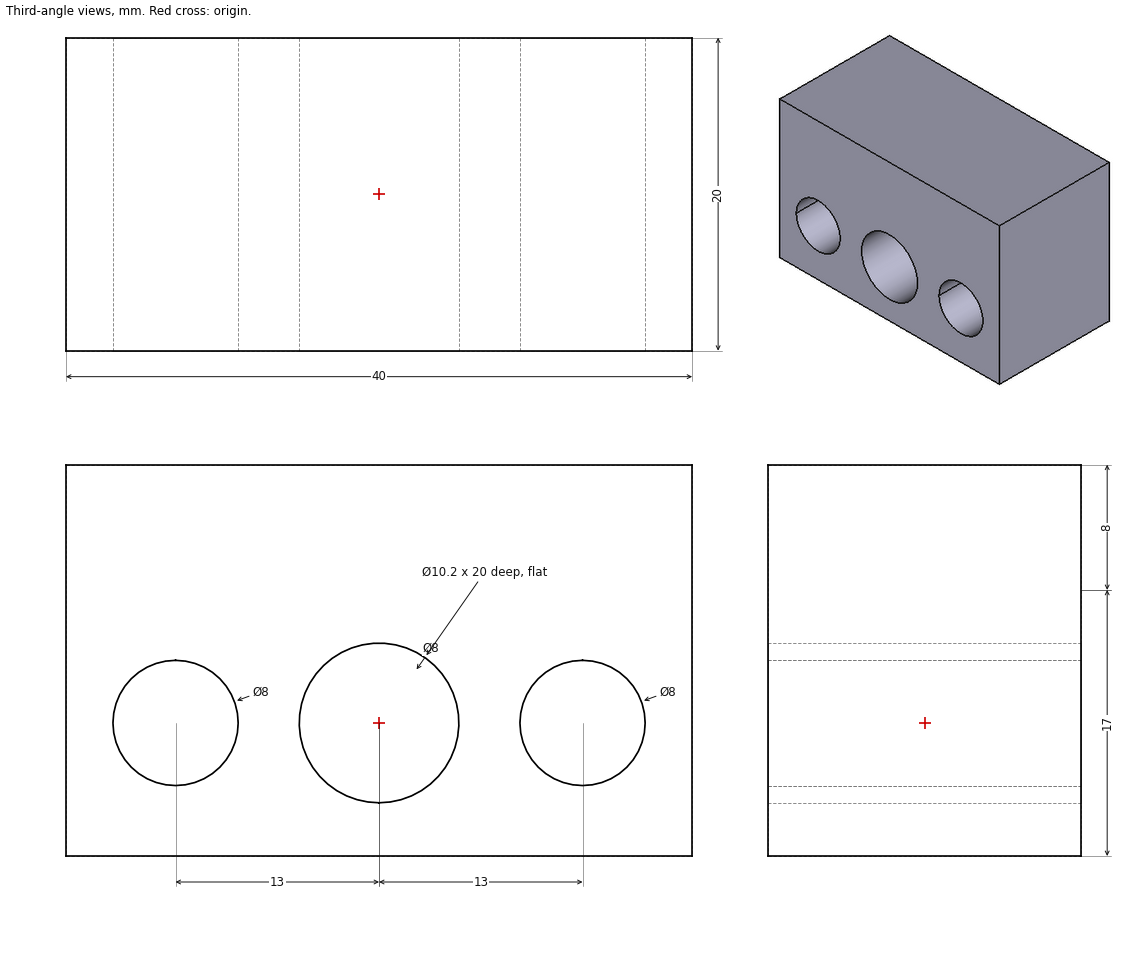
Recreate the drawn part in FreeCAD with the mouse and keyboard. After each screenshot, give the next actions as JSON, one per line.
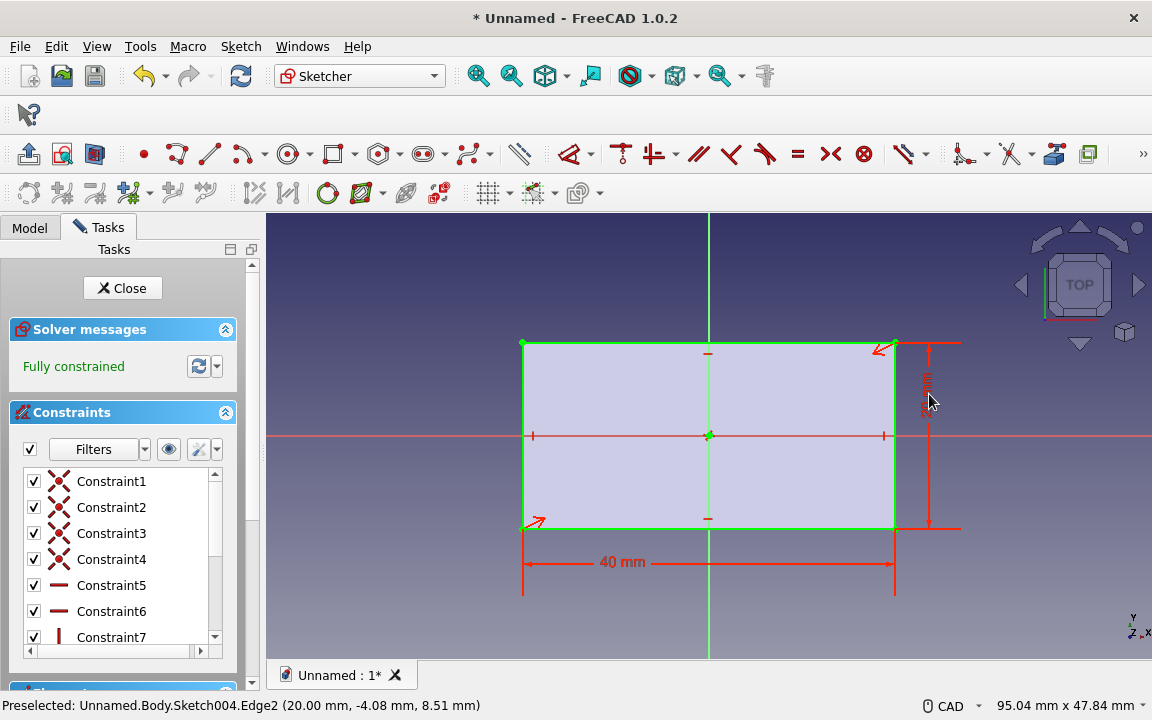
{"action": "left_click", "coordinate": [123, 288]}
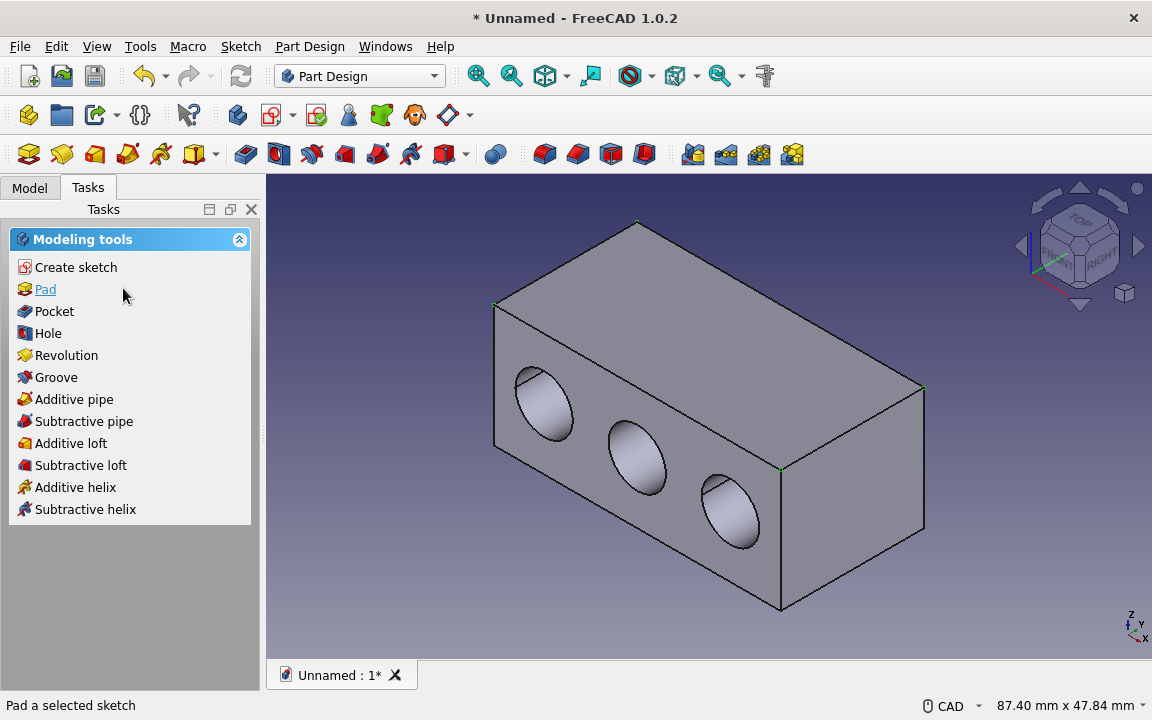
{"action": "left_click", "coordinate": [29, 154]}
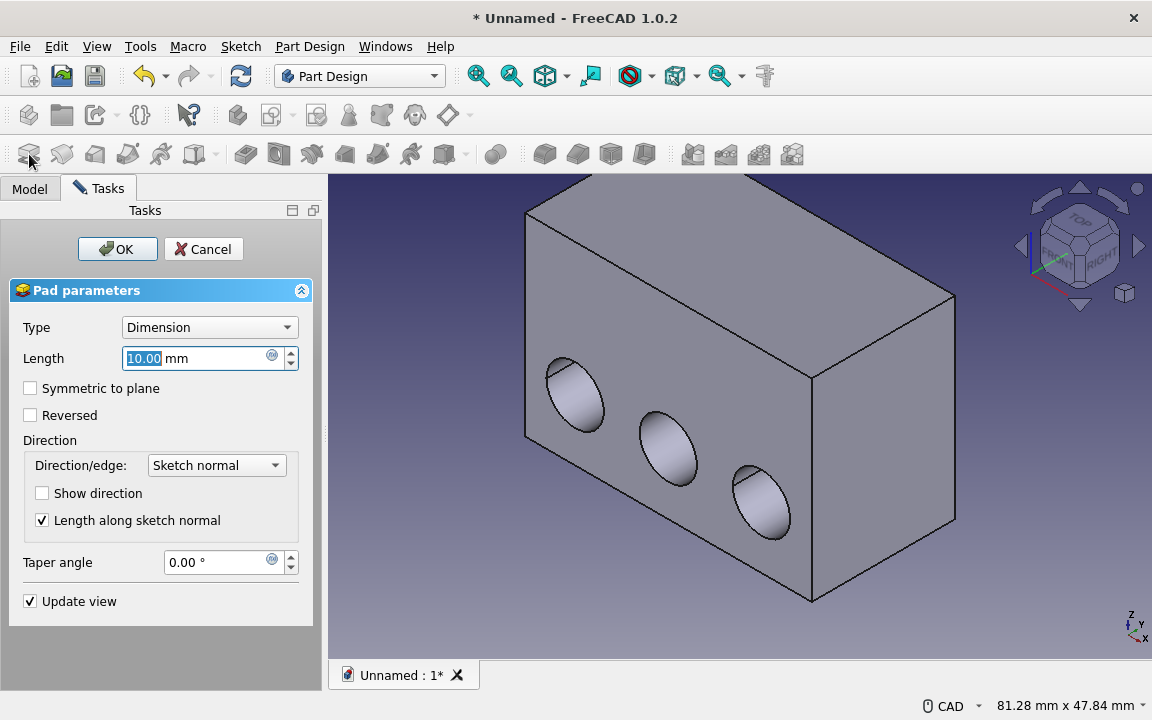
{"action": "type", "text": "8"}
{"action": "key", "text": "Tab"}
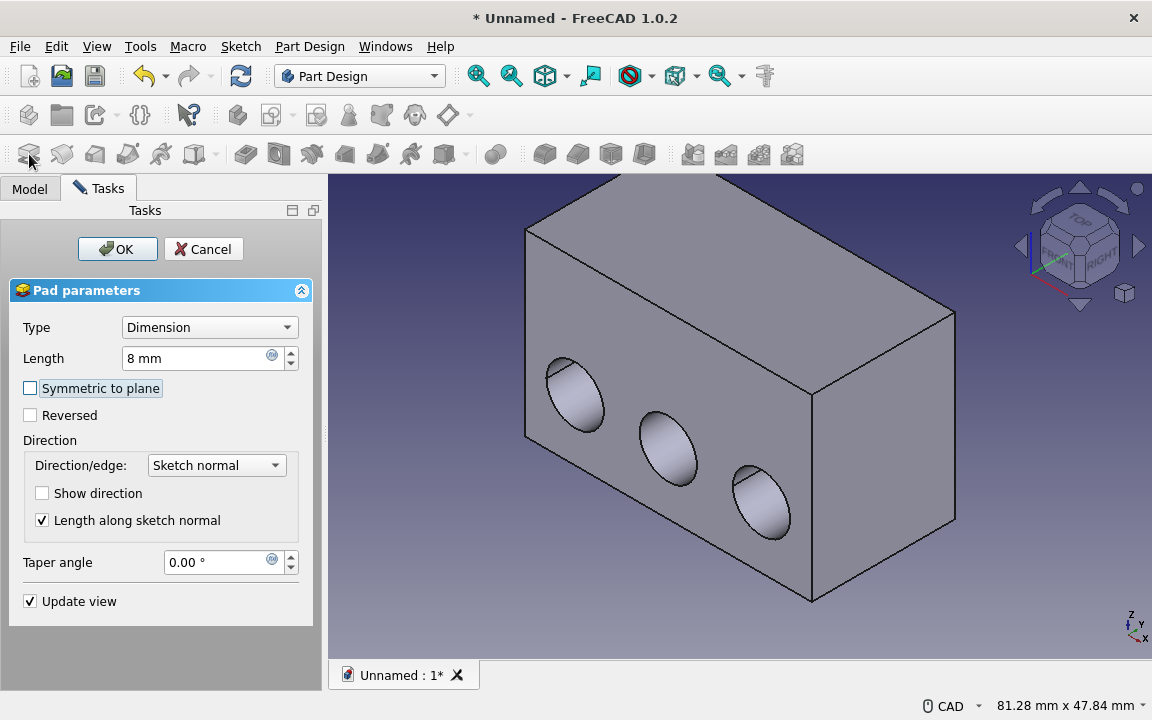
{"action": "left_click", "coordinate": [118, 249]}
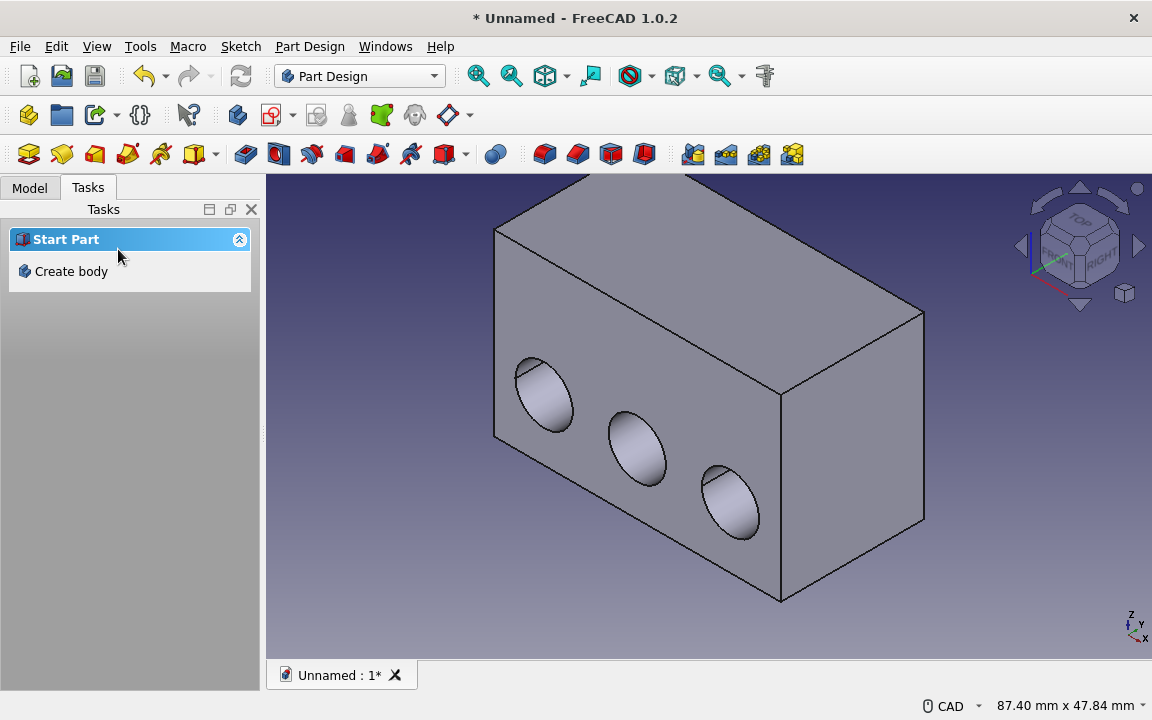
{"action": "left_click", "coordinate": [479, 76]}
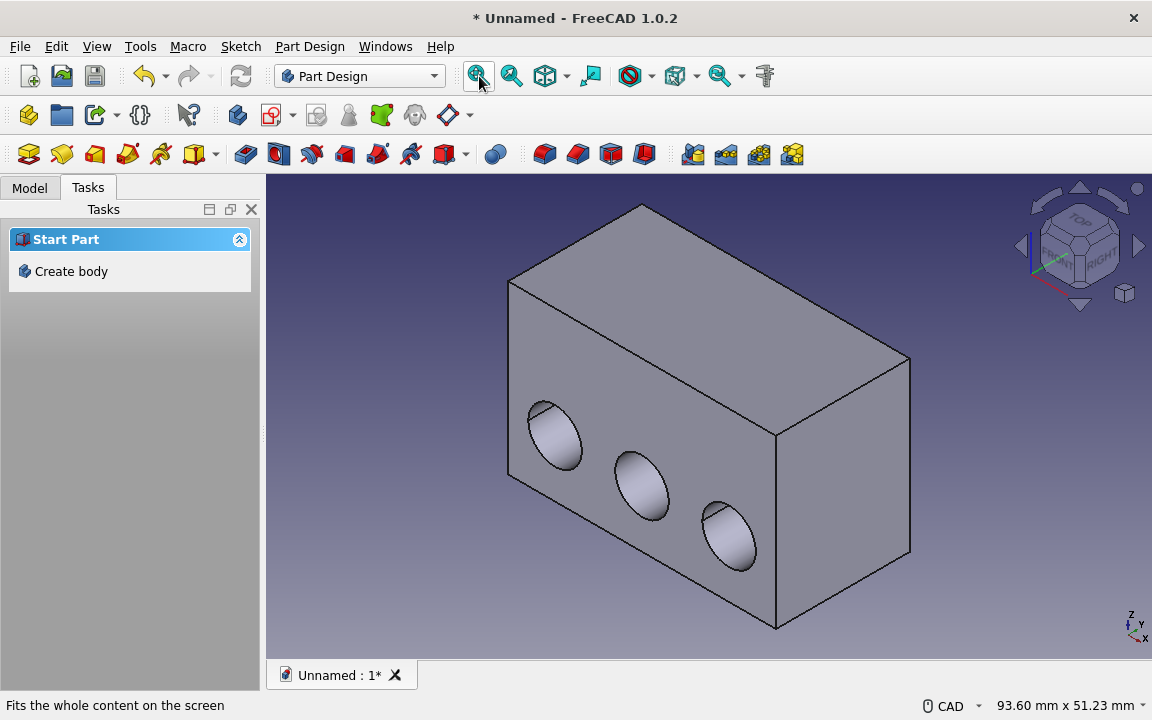
{"action": "key", "text": "4"}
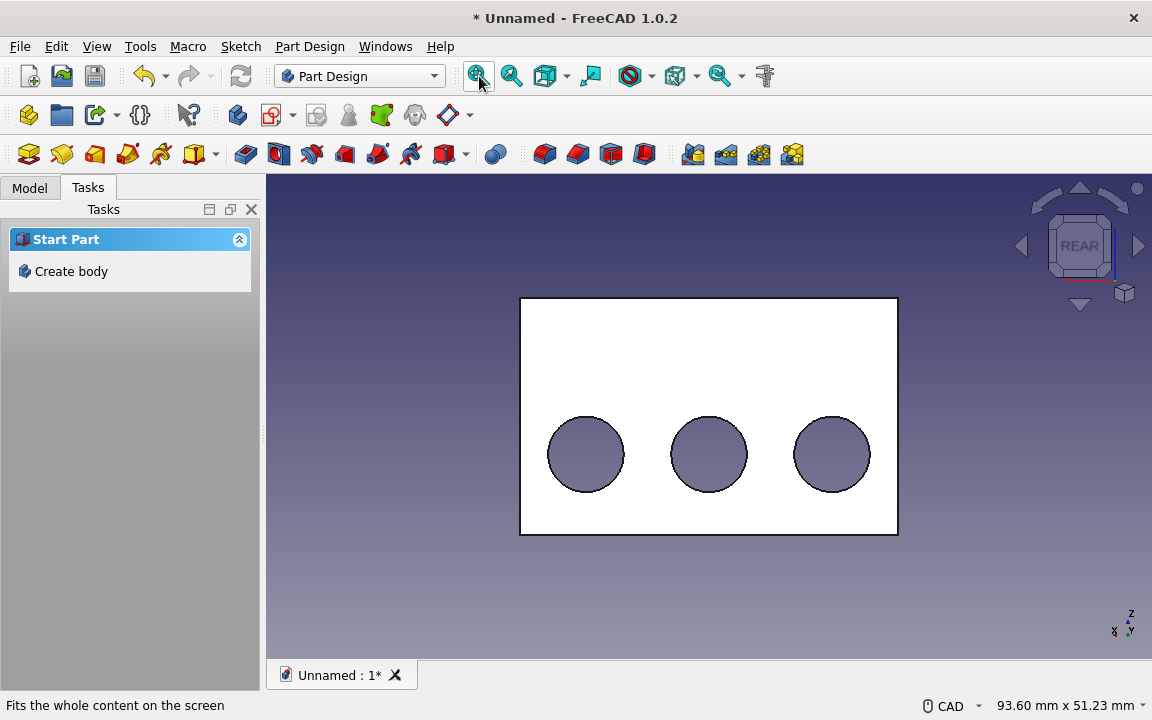
{"action": "left_click", "coordinate": [655, 382]}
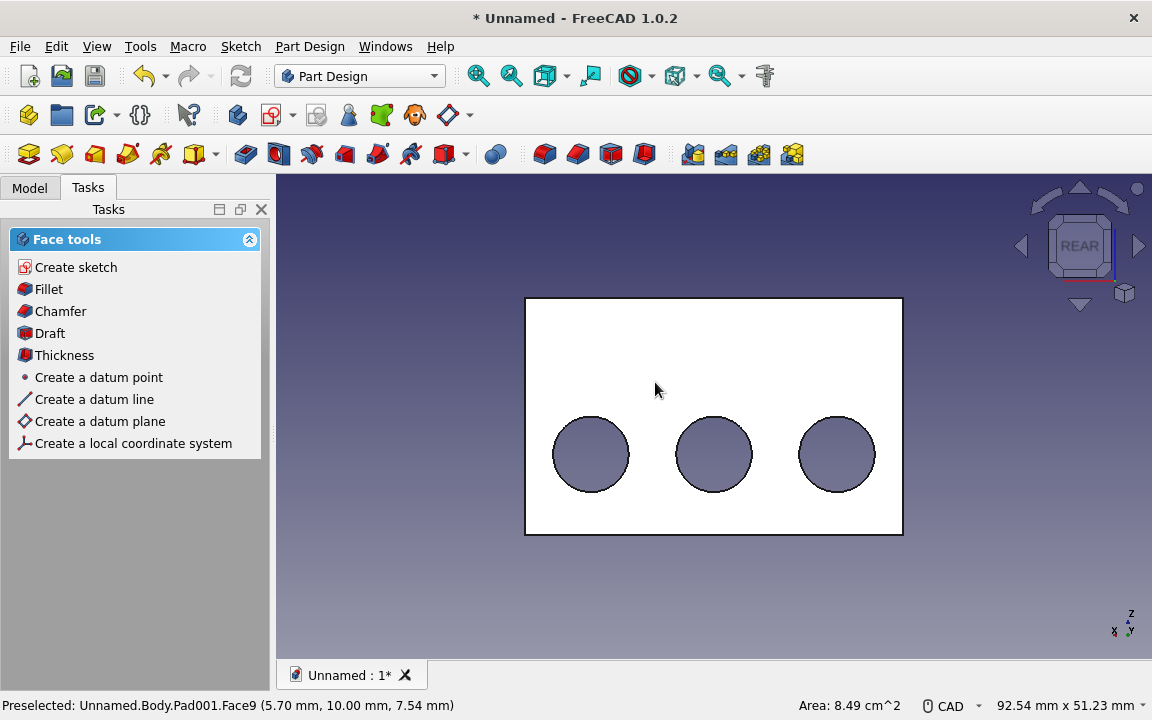
{"action": "left_click", "coordinate": [270, 116]}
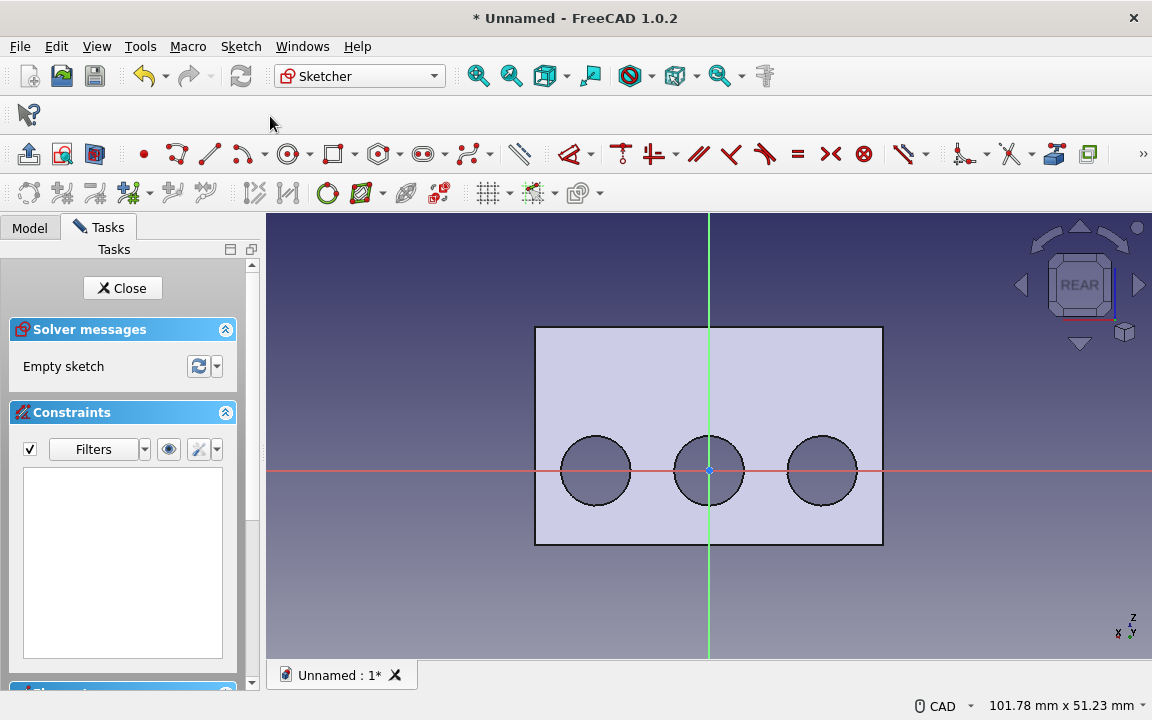
{"action": "scroll", "coordinate": [739, 486], "scroll_direction": "up", "scroll_amount": 6}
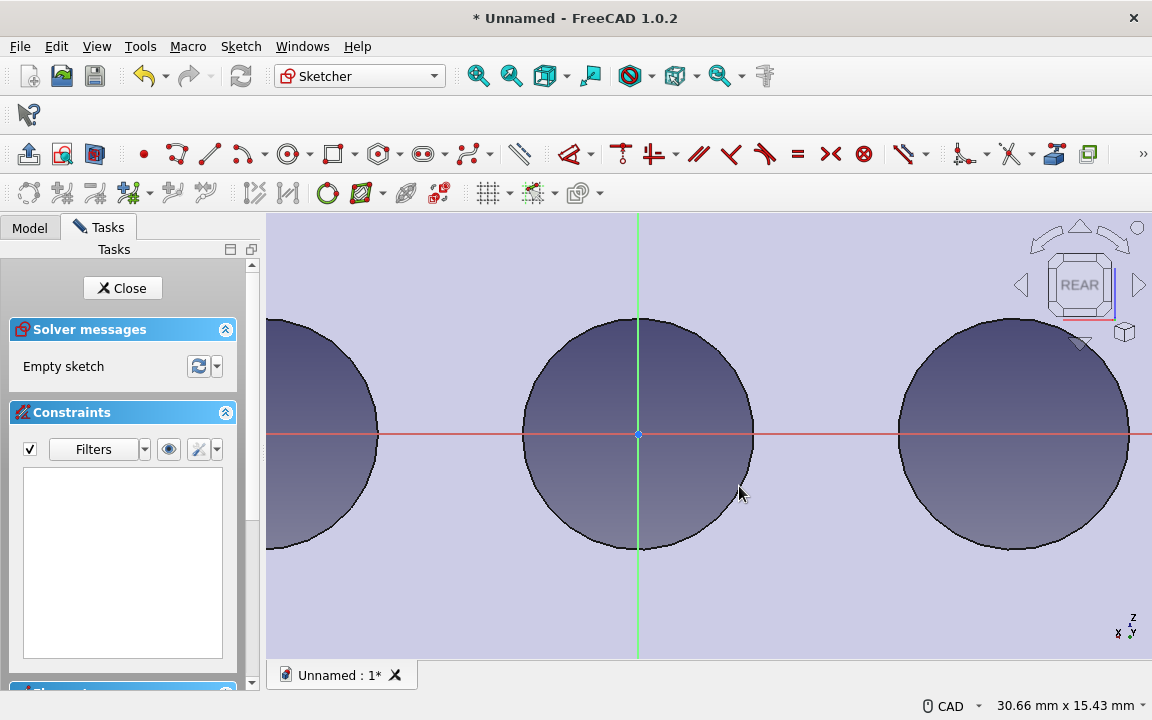
{"action": "left_click", "coordinate": [288, 154]}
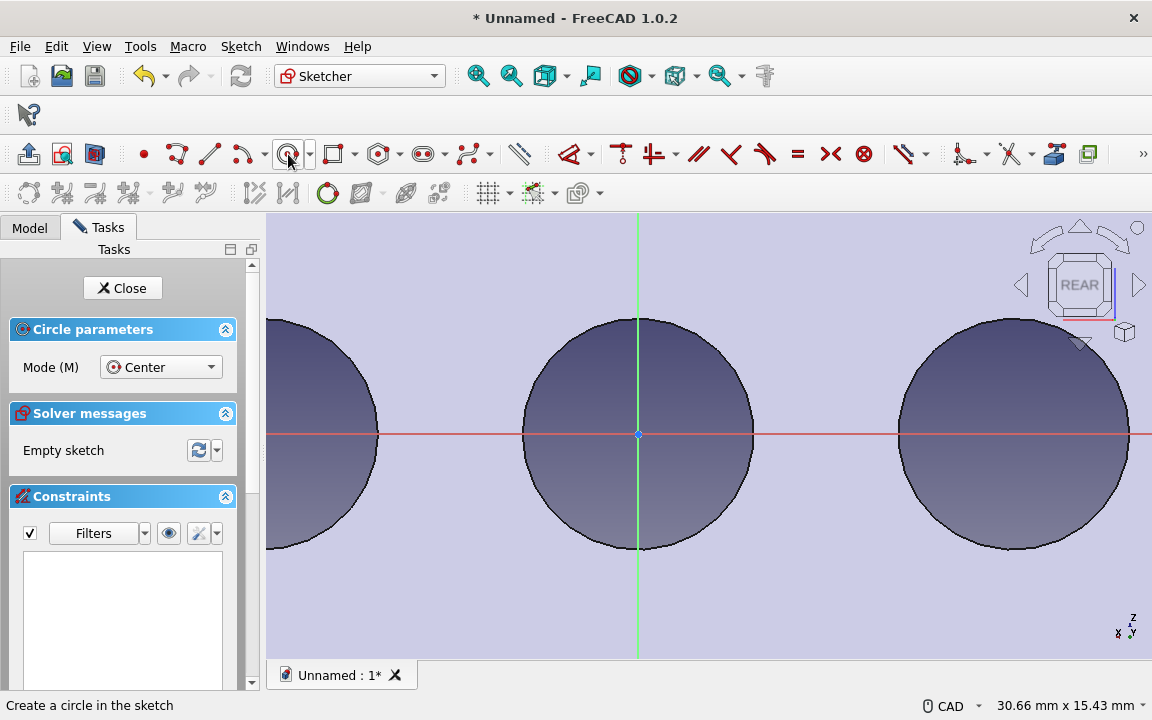
{"action": "left_click", "coordinate": [638, 434]}
{"action": "left_click", "coordinate": [742, 330]}
{"action": "key", "text": "Escape"}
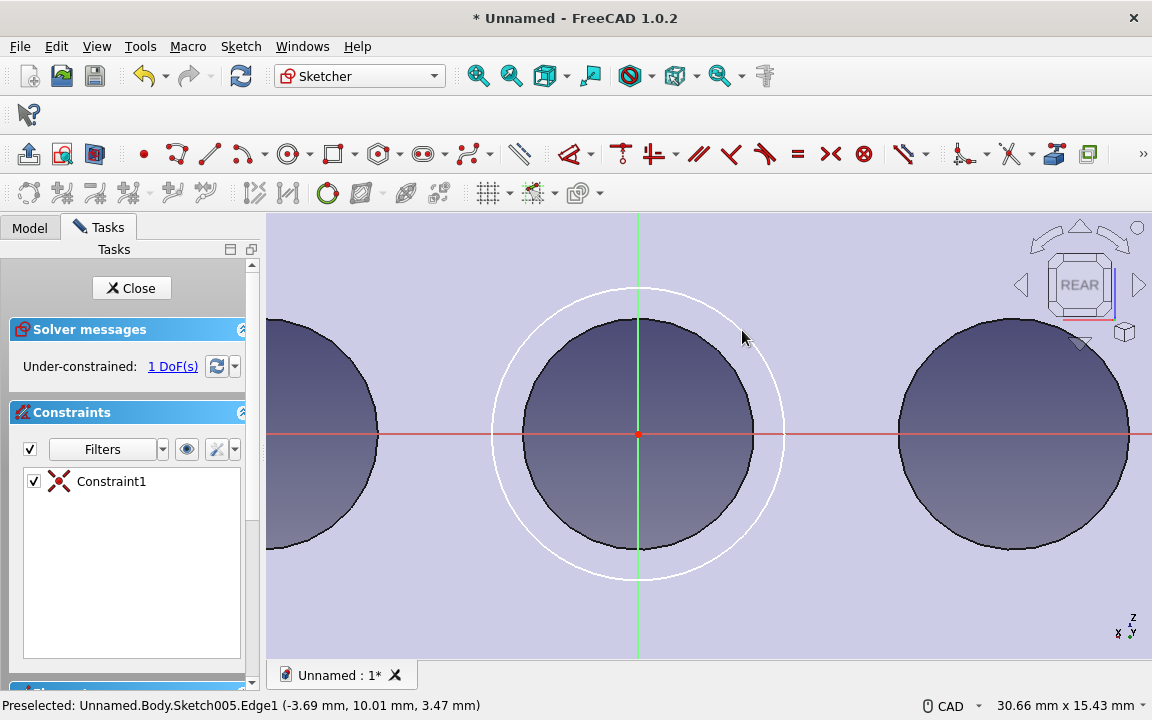
{"action": "left_click", "coordinate": [568, 154]}